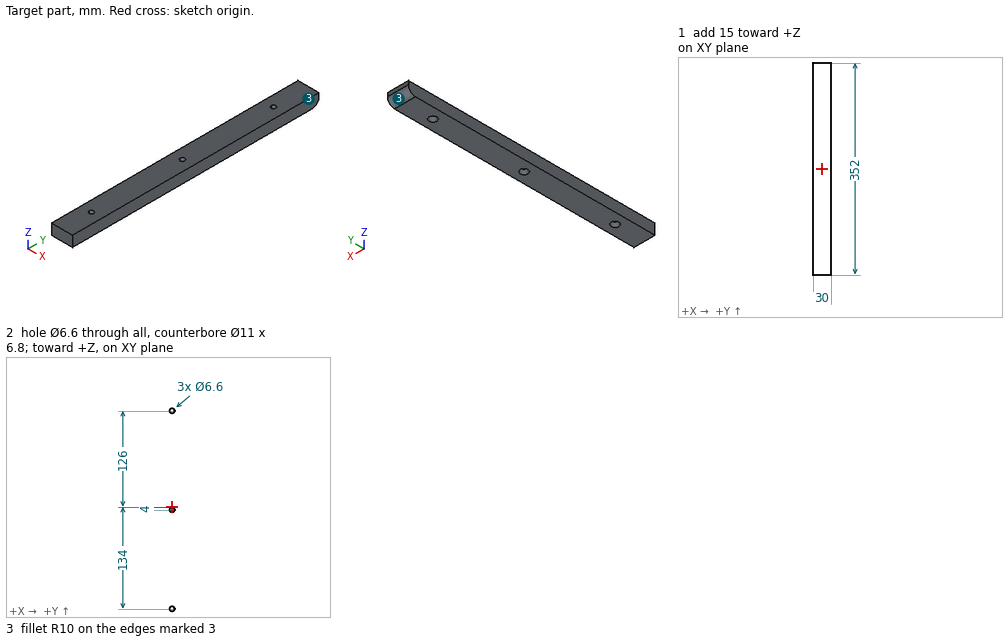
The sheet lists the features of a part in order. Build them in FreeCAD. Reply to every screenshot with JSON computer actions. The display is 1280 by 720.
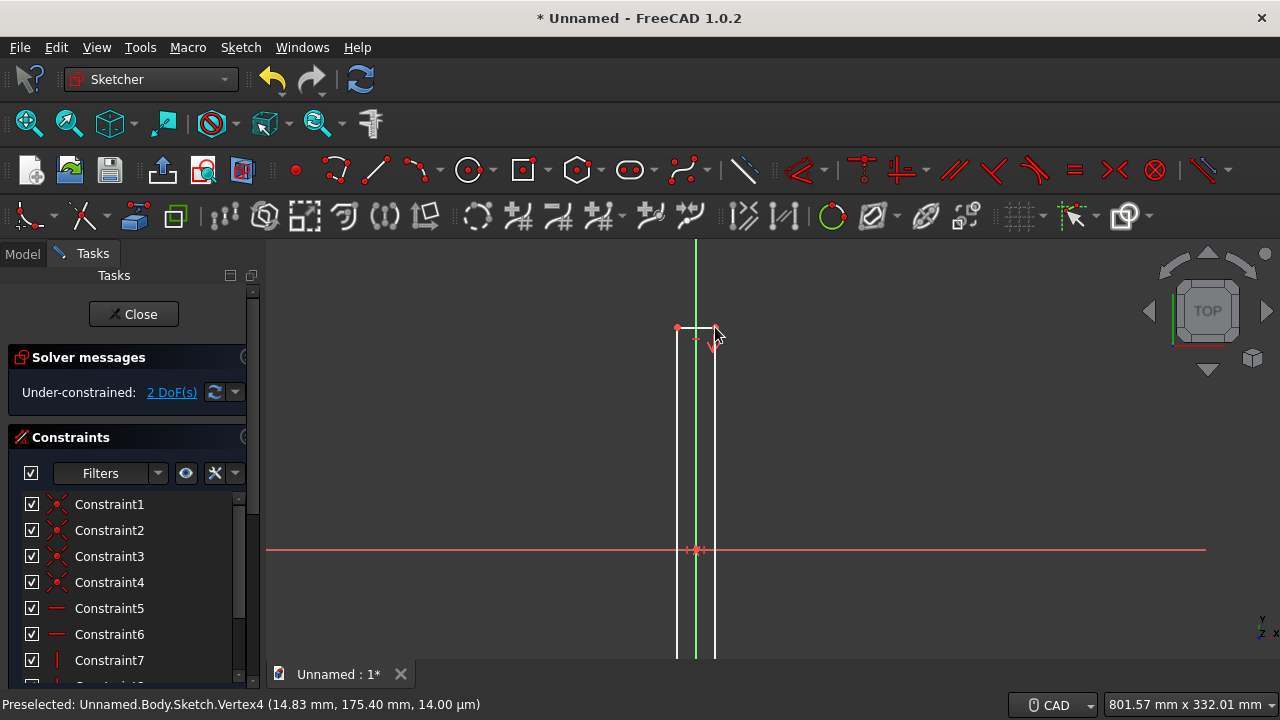
{"action": "left_click", "coordinate": [800, 170]}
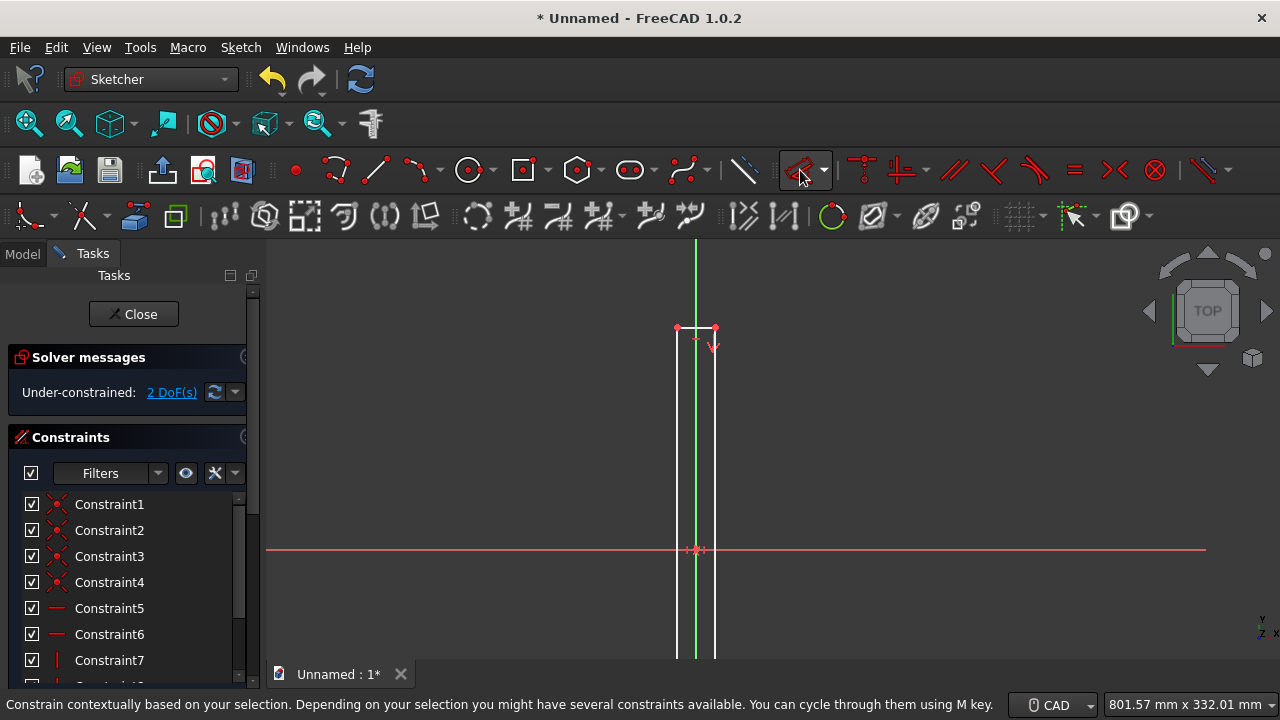
{"action": "scroll", "coordinate": [715, 326], "scroll_direction": "down", "scroll_amount": 3}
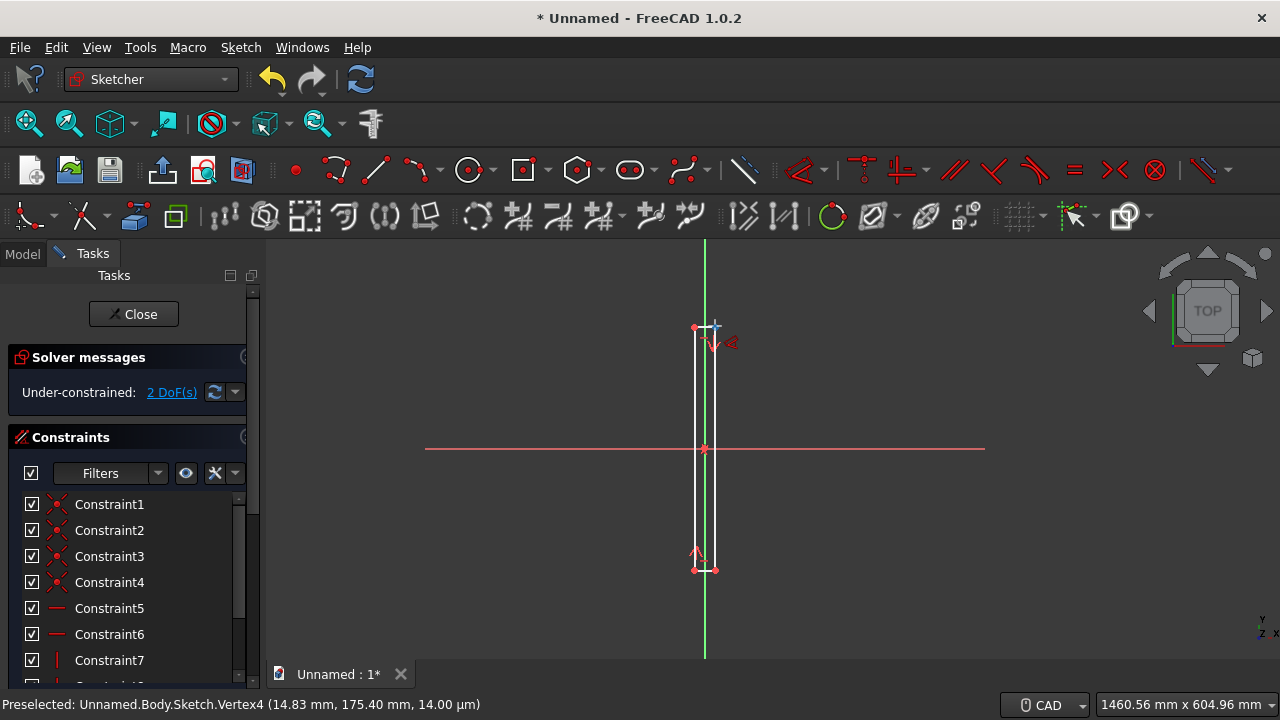
{"action": "scroll", "coordinate": [703, 571], "scroll_direction": "up", "scroll_amount": 4}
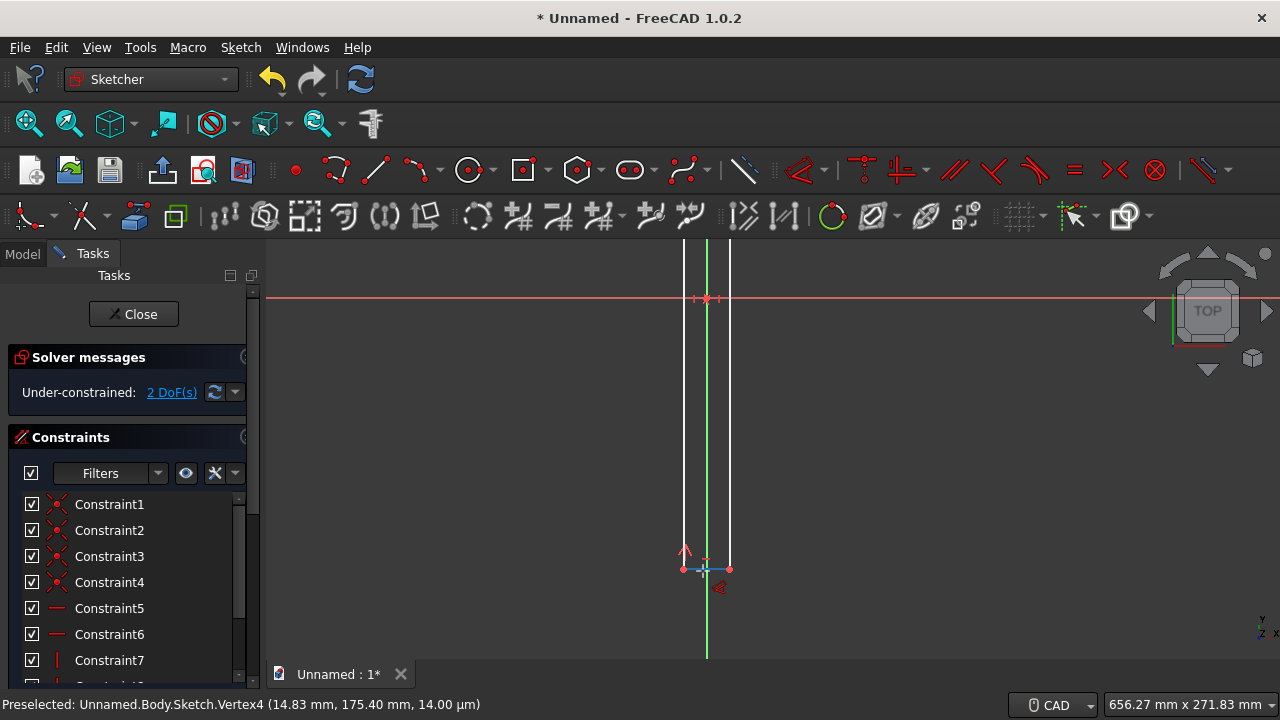
{"action": "left_click", "coordinate": [702, 569]}
{"action": "left_click", "coordinate": [691, 603]}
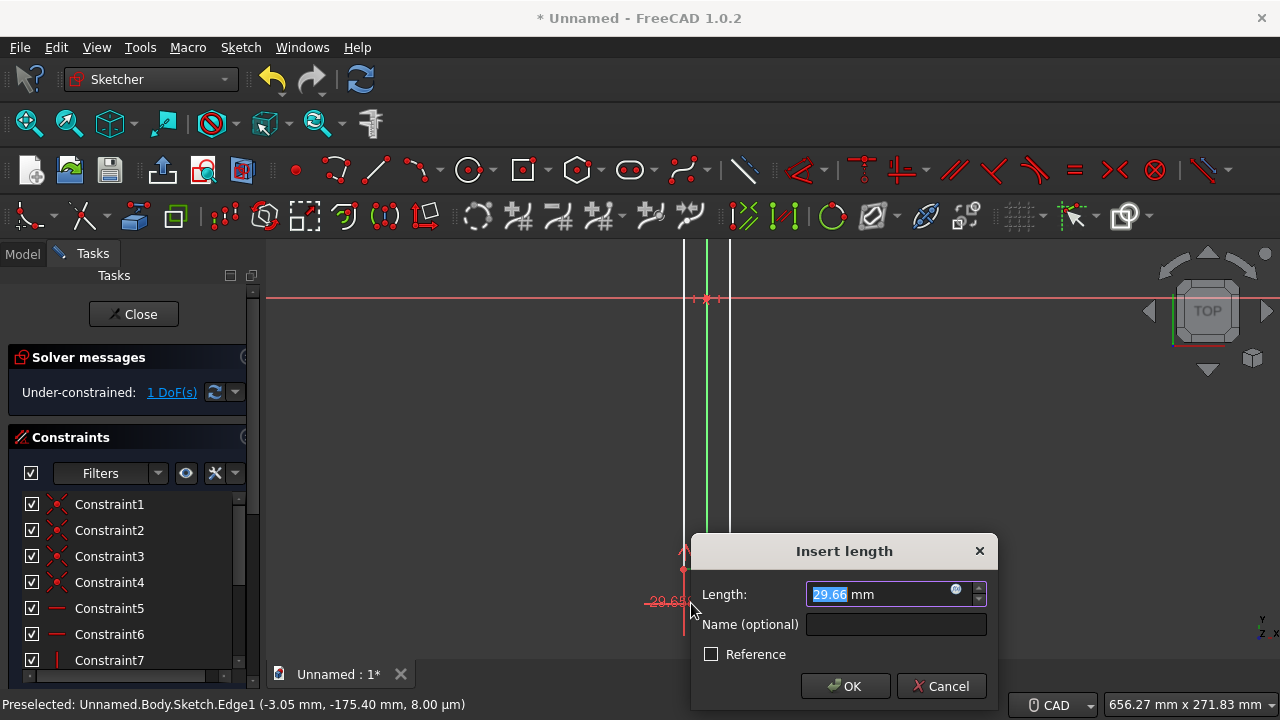
{"action": "type", "text": "30"}
{"action": "key", "text": "Return"}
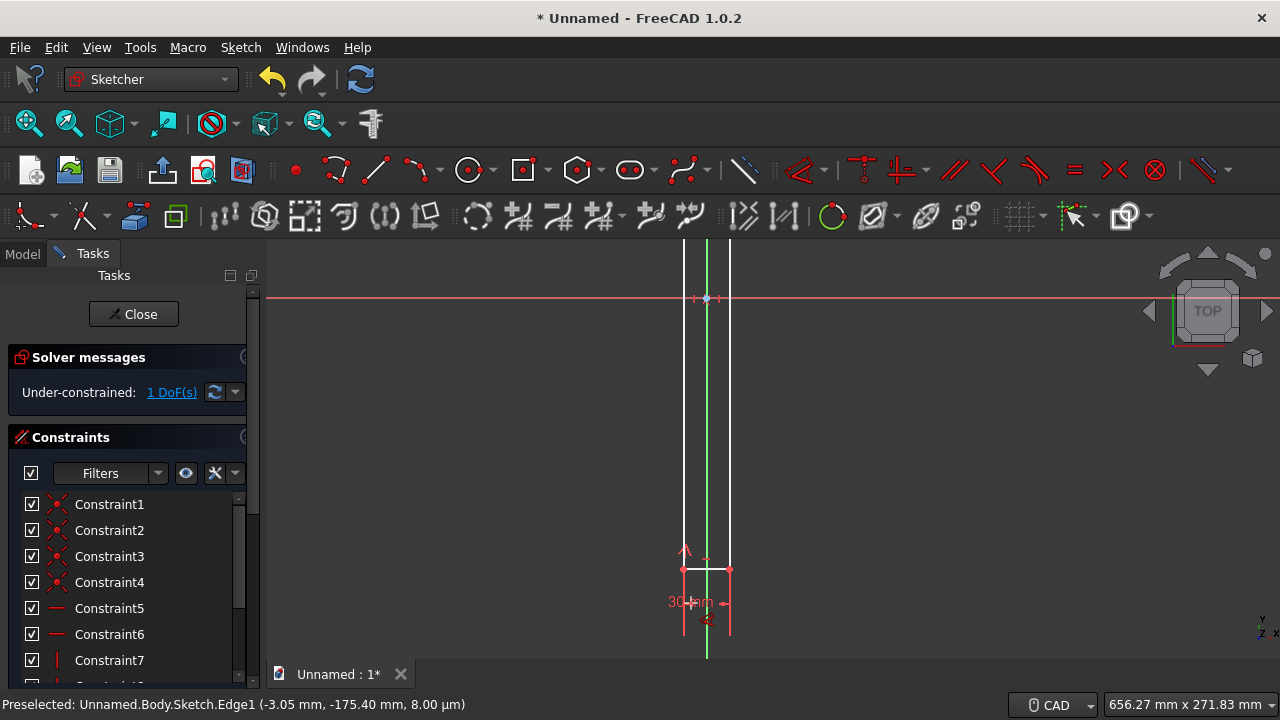
{"action": "left_click", "coordinate": [730, 407]}
{"action": "left_click", "coordinate": [764, 418]}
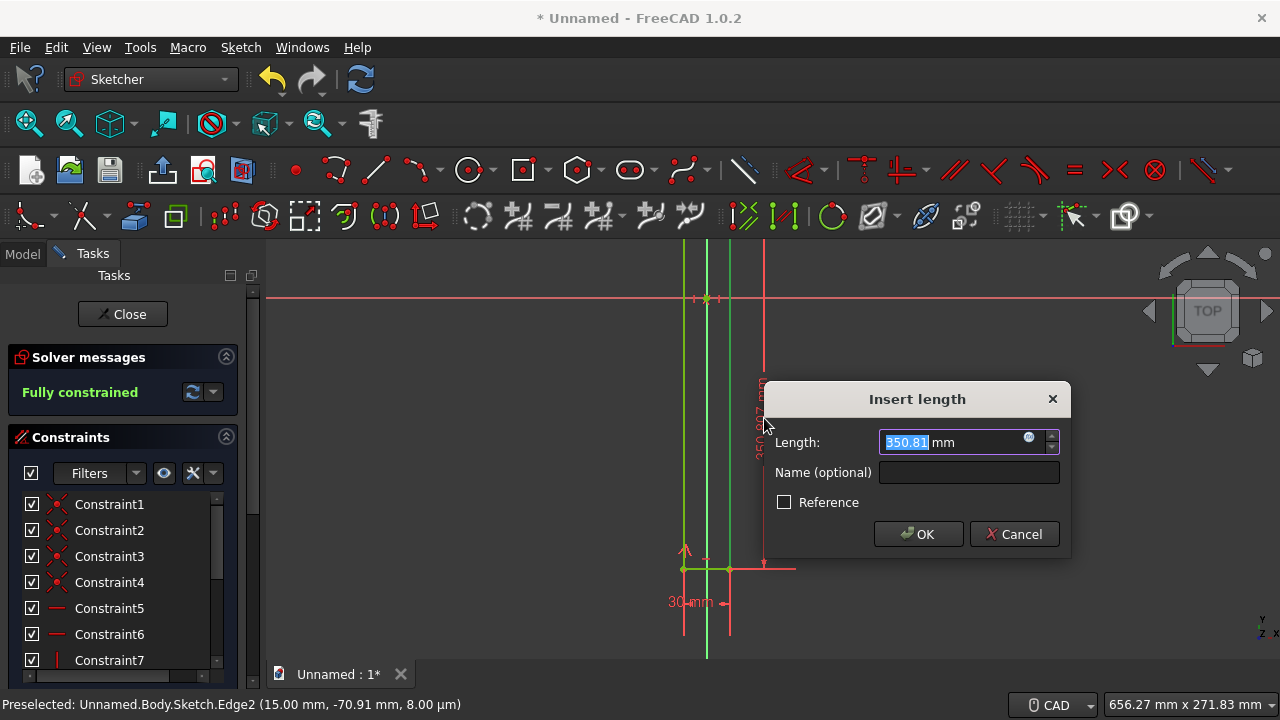
{"action": "type", "text": "352"}
{"action": "key", "text": "Return"}
{"action": "key", "text": "Escape"}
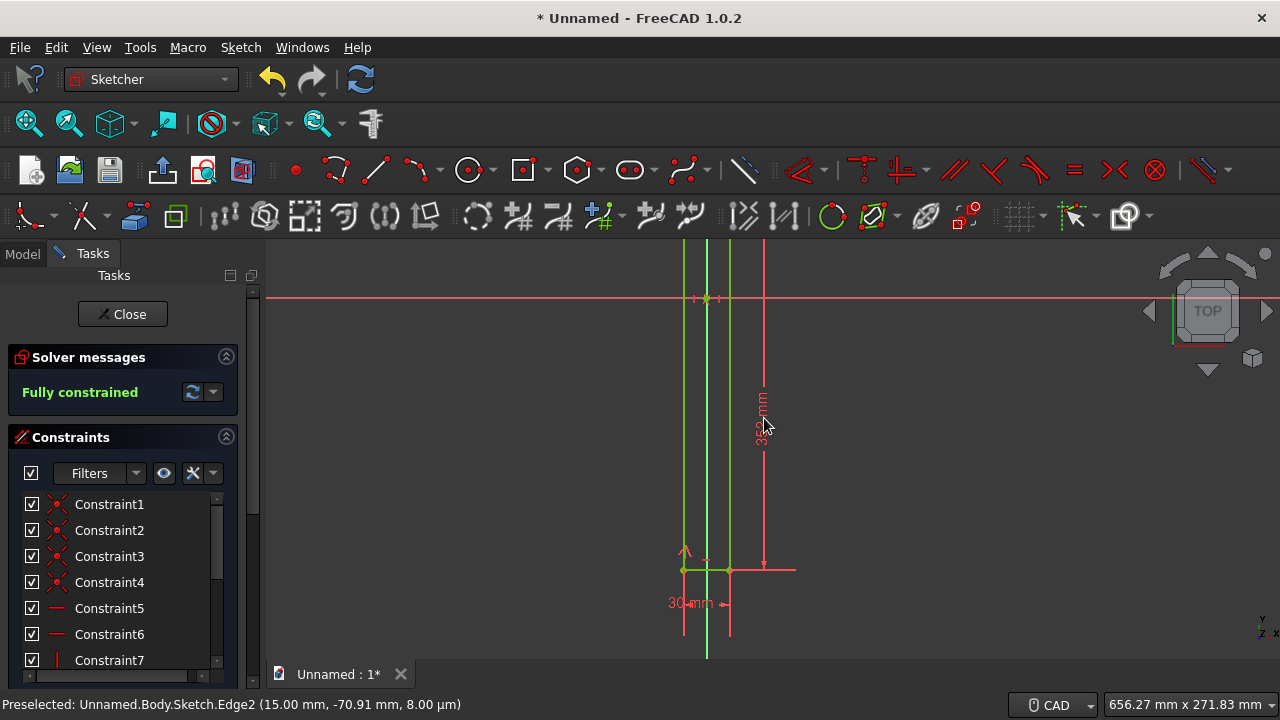
{"action": "left_click", "coordinate": [123, 314]}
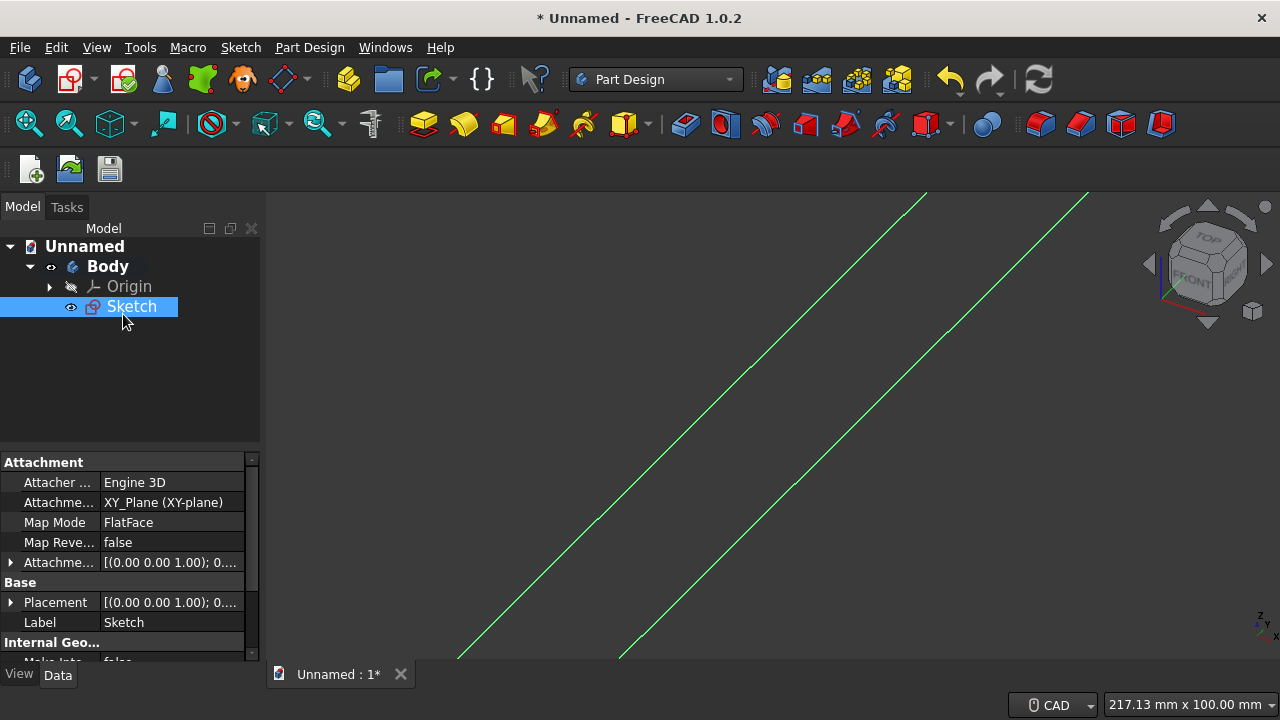
{"action": "left_click", "coordinate": [424, 124]}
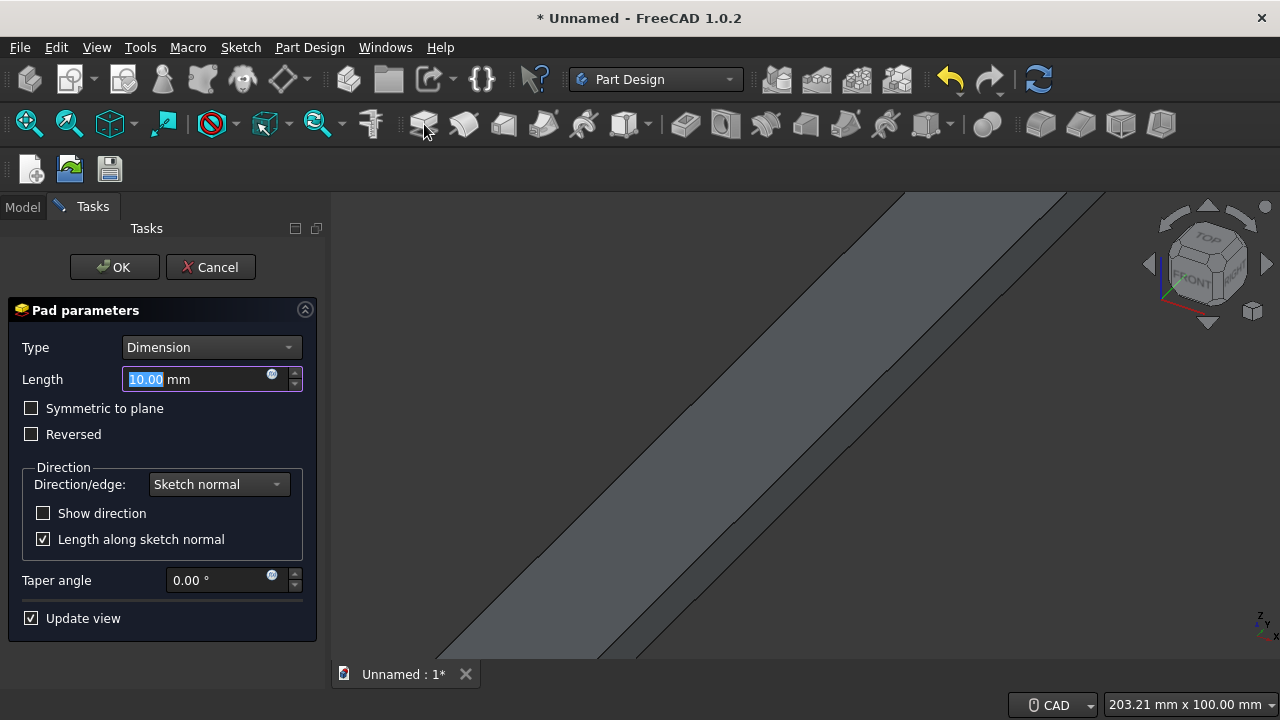
{"action": "type", "text": "15"}
{"action": "key", "text": "Tab"}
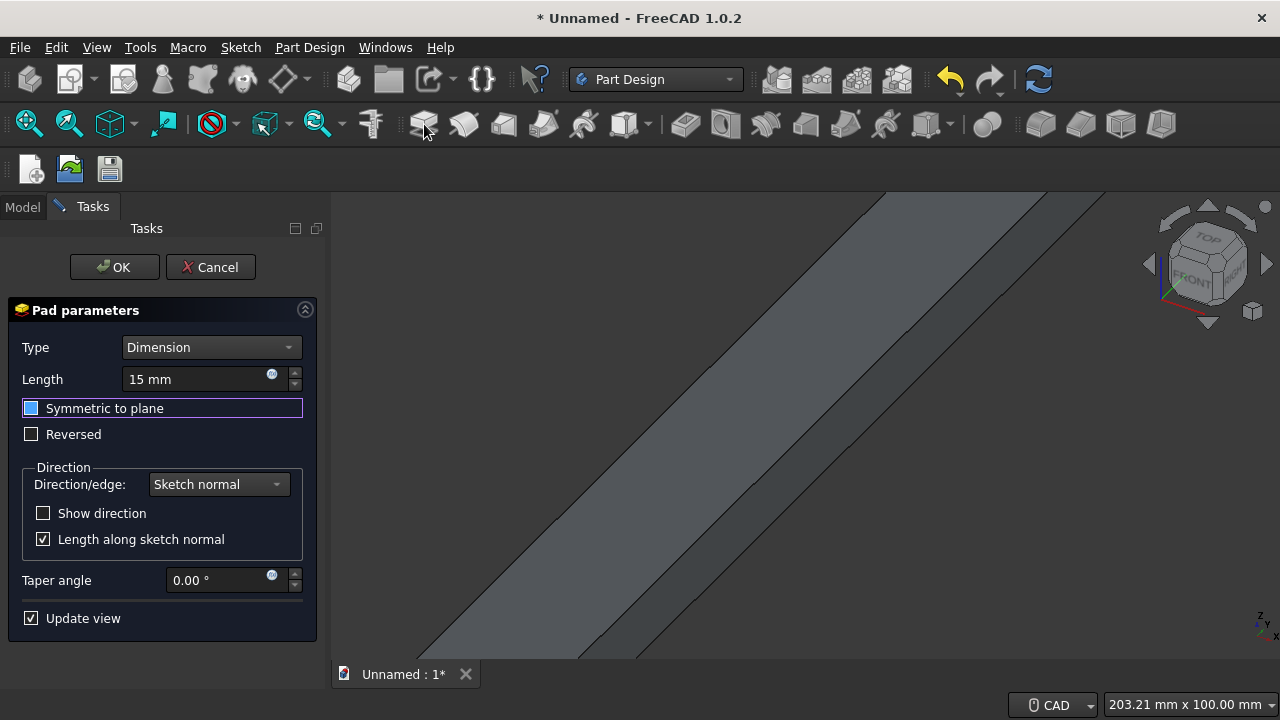
{"action": "left_click", "coordinate": [115, 267]}